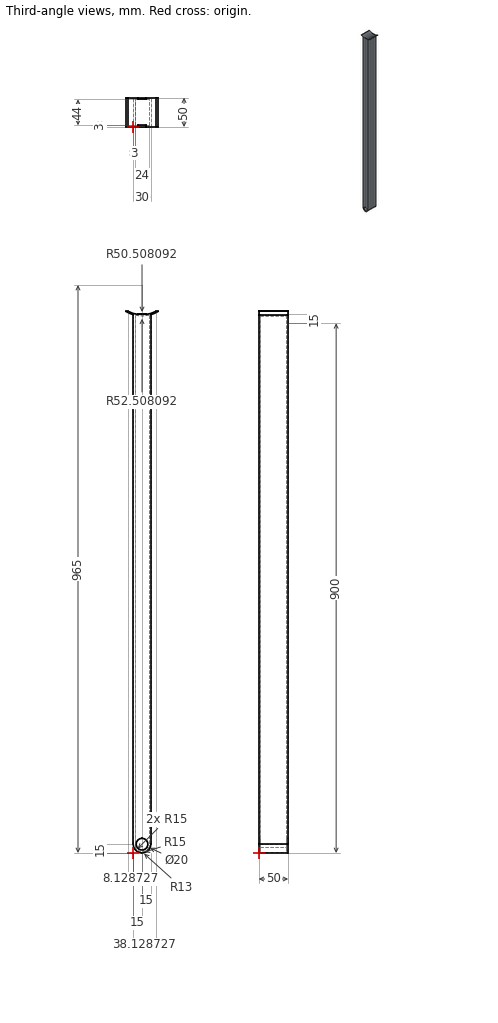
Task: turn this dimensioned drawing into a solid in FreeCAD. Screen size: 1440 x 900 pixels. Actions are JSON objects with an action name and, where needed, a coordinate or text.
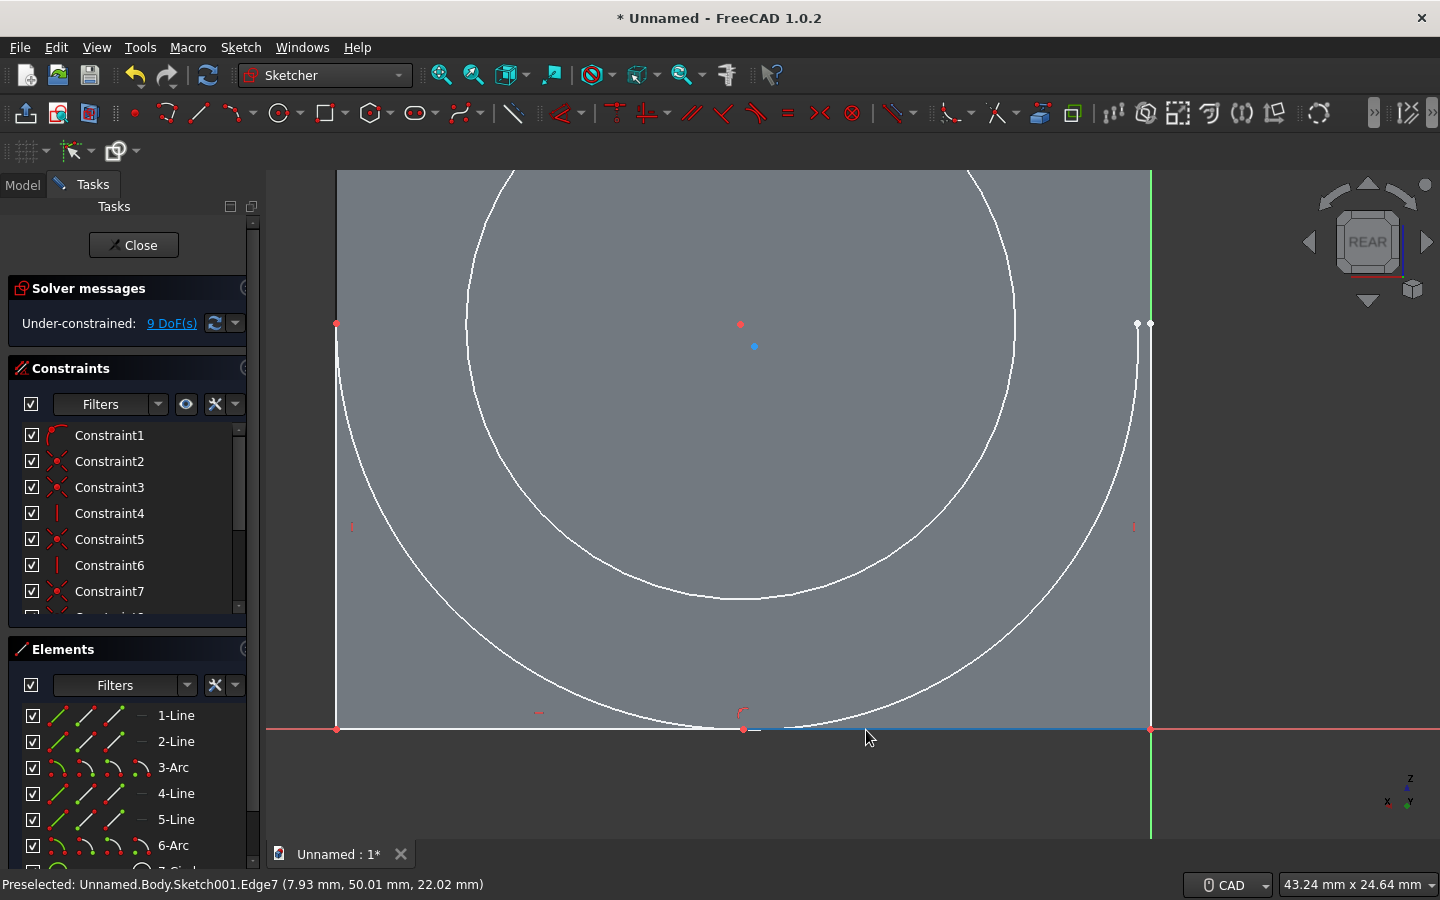
{"action": "left_click", "coordinate": [866, 729]}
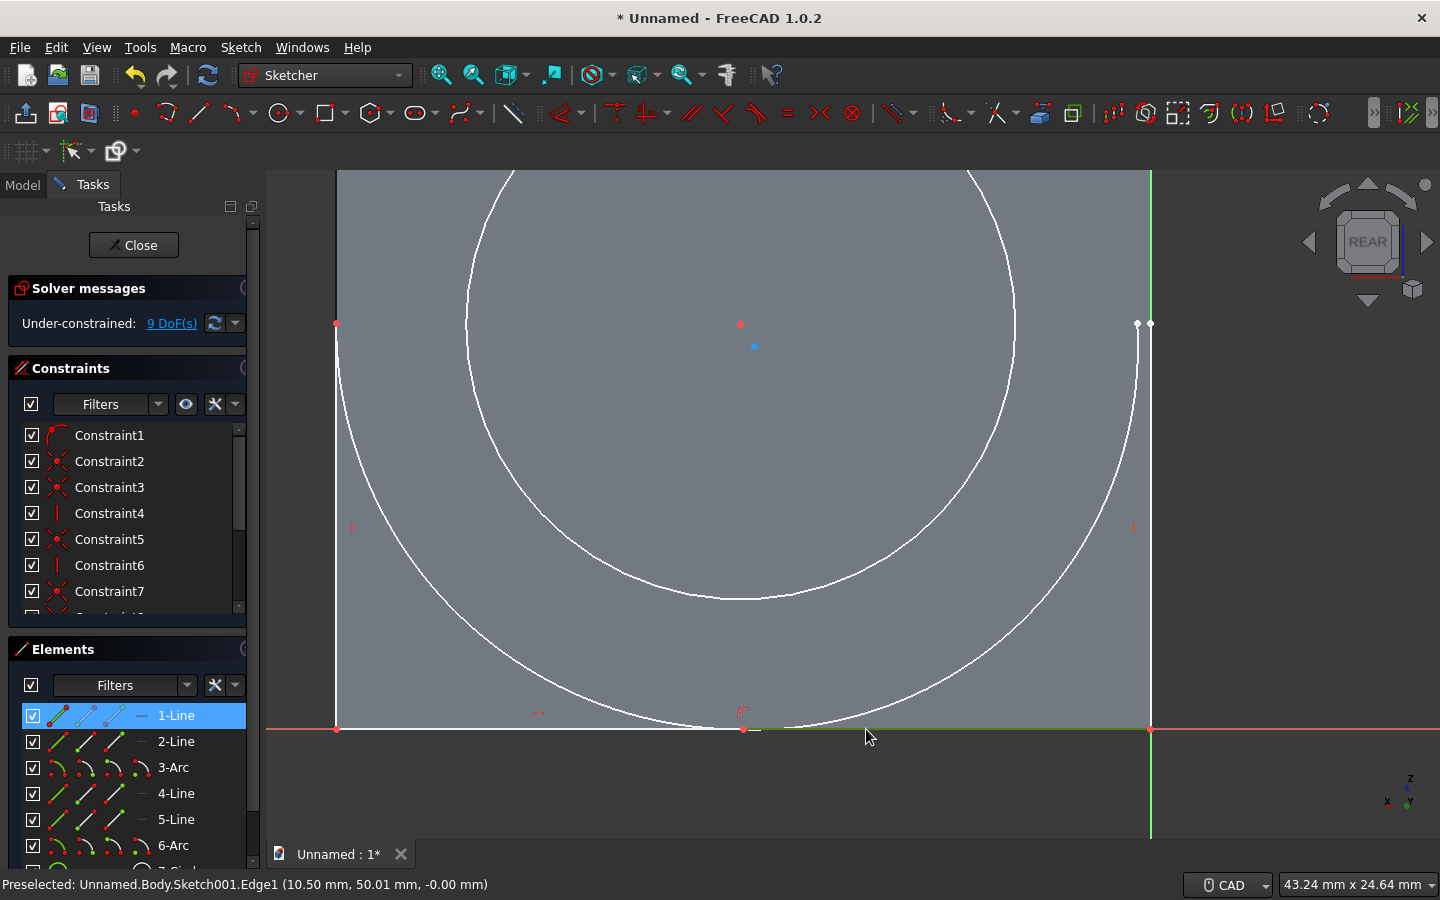
{"action": "left_click", "coordinate": [928, 688]}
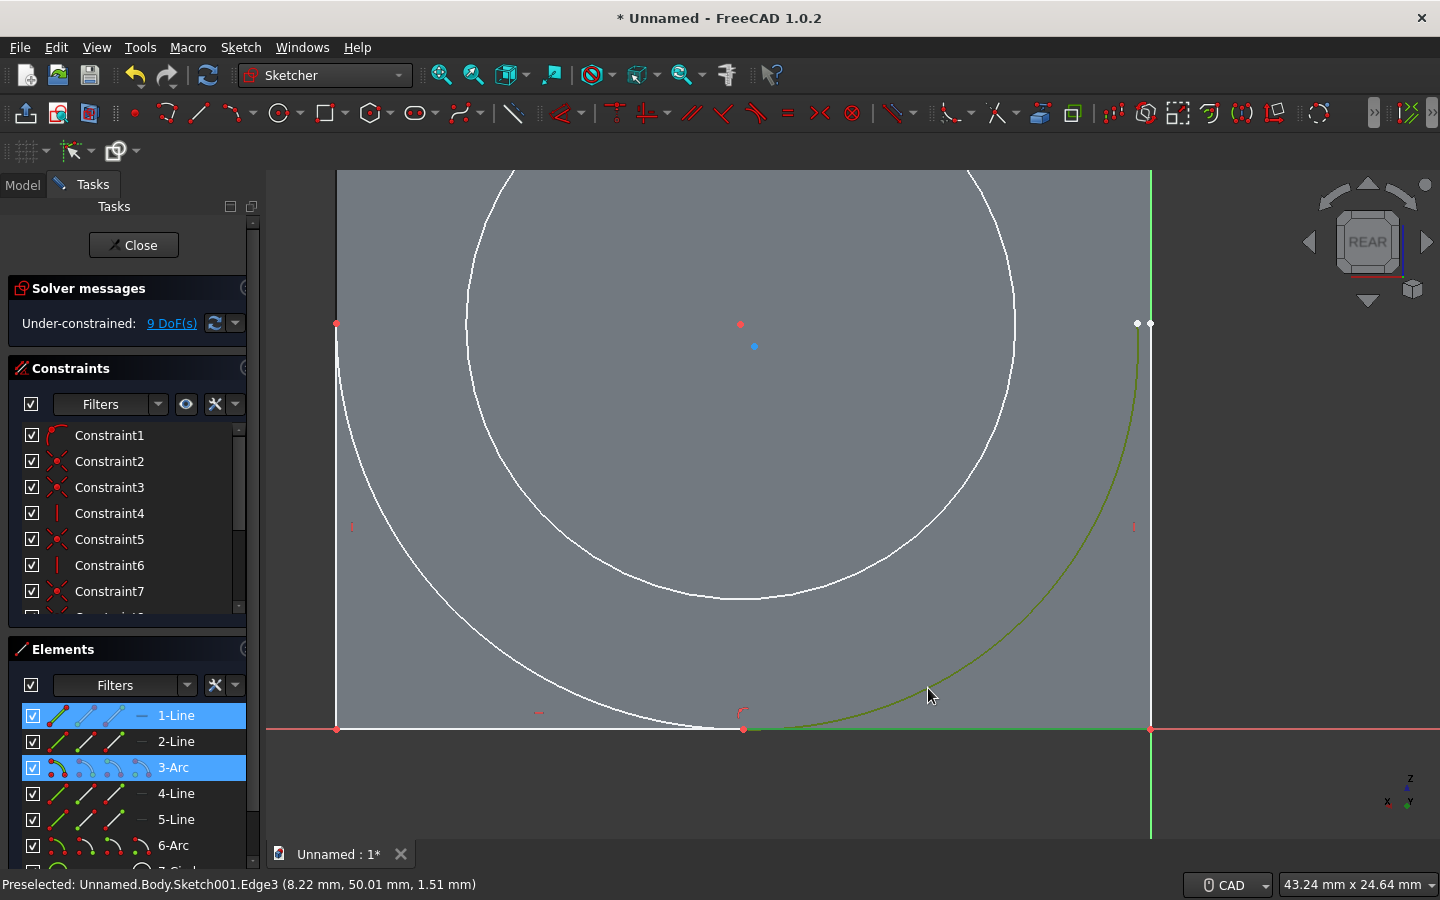
{"action": "left_click", "coordinate": [756, 114]}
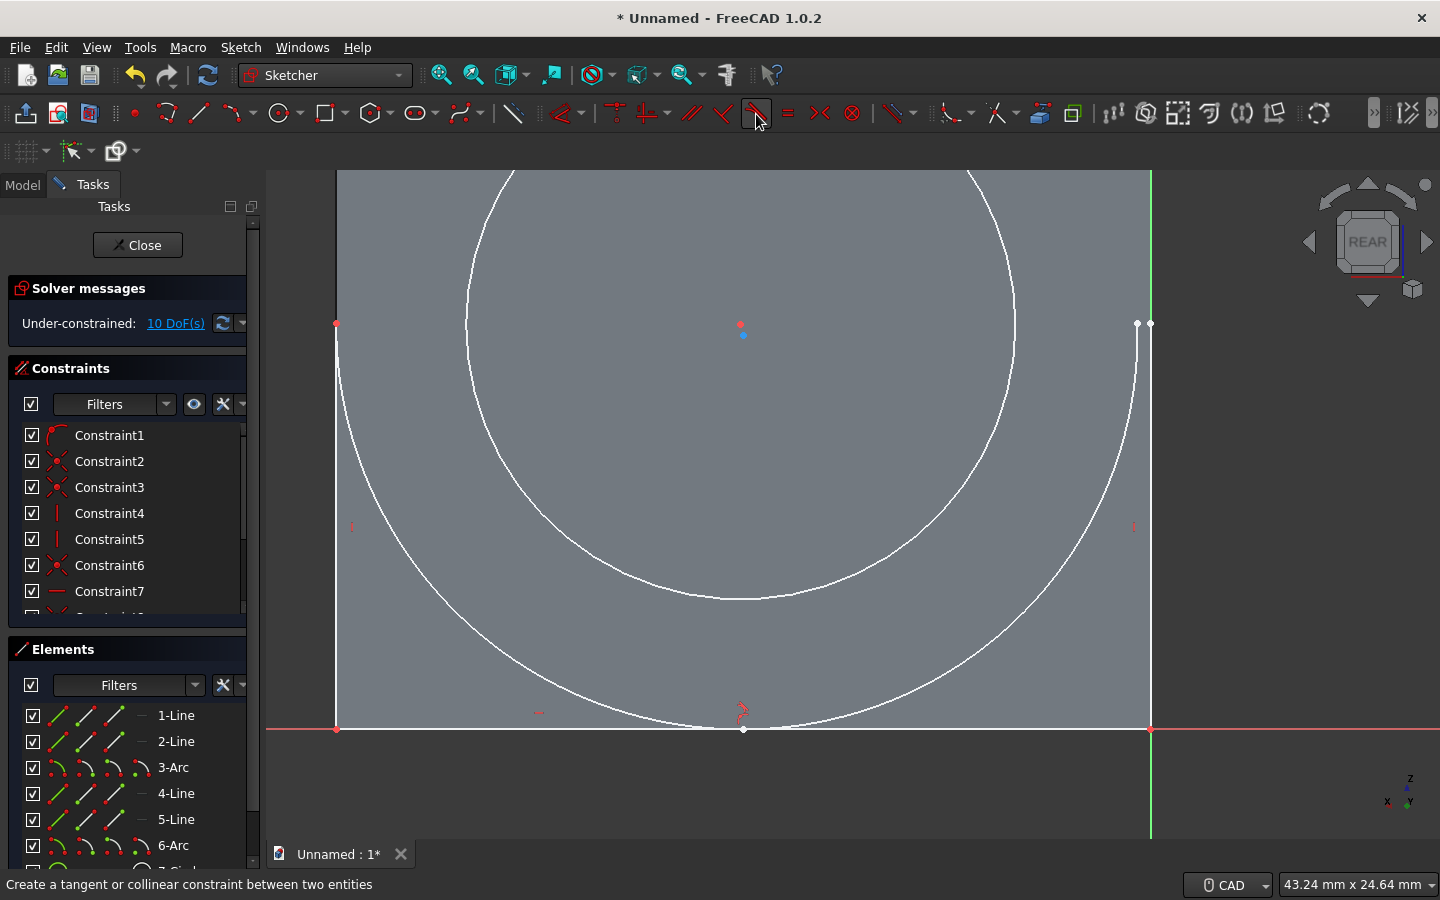
{"action": "left_click", "coordinate": [866, 729]}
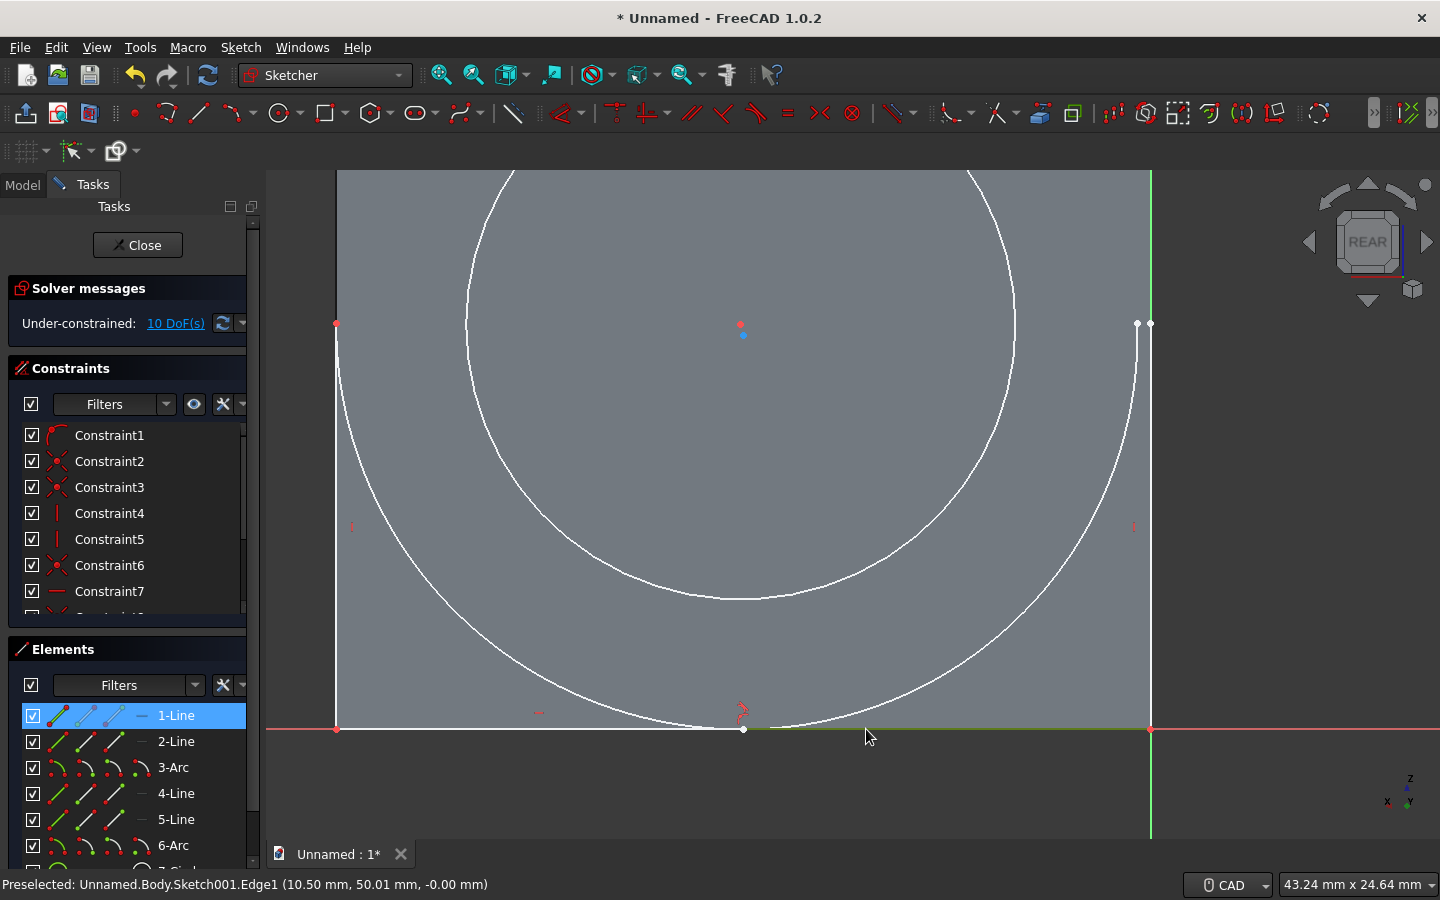
{"action": "left_click", "coordinate": [380, 509]}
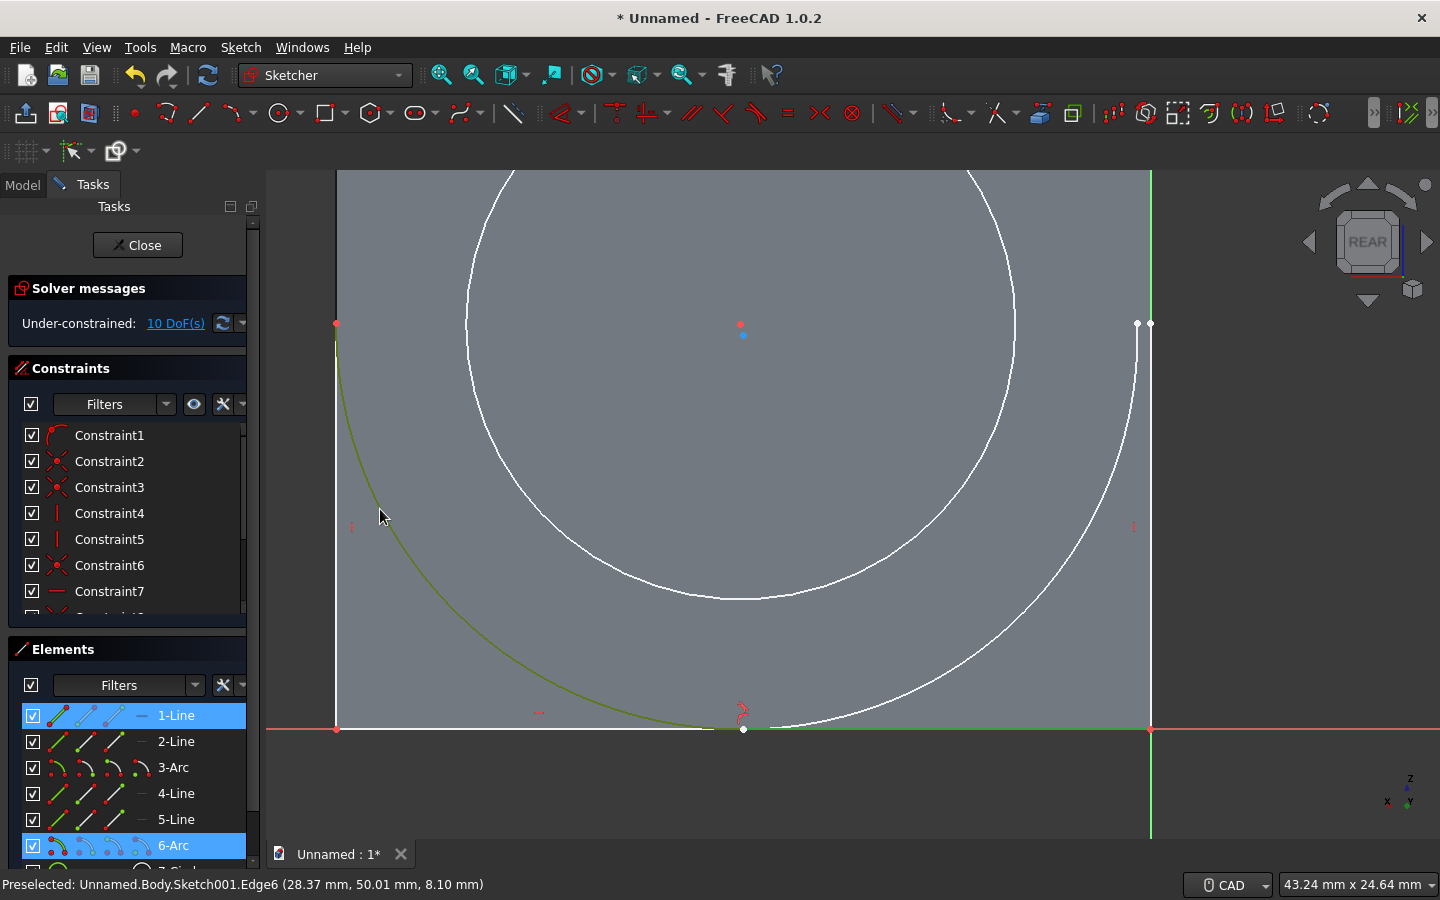
{"action": "left_click", "coordinate": [756, 114]}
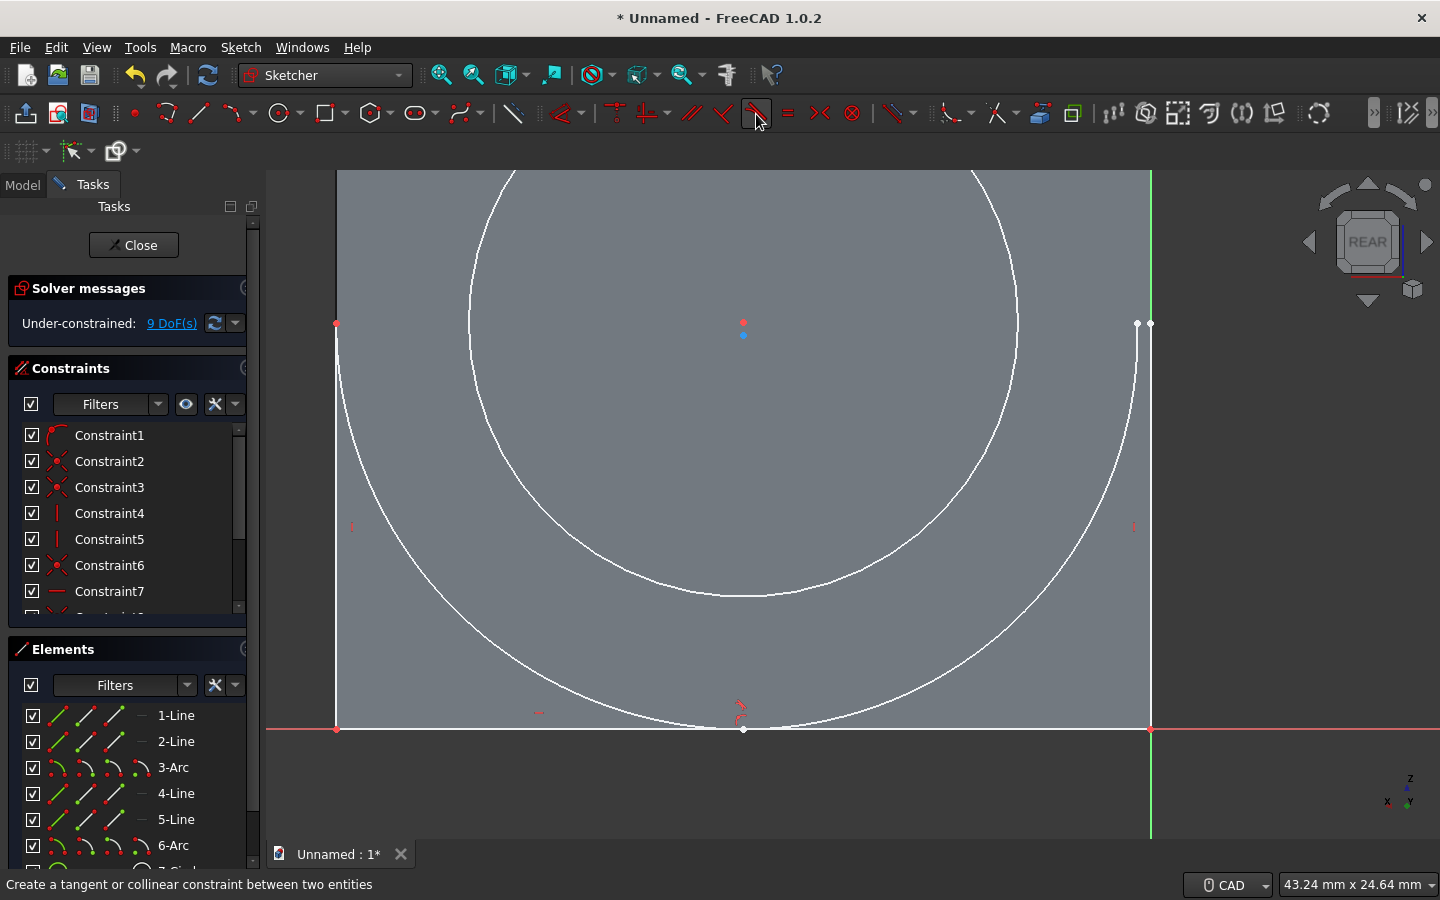
{"action": "left_click", "coordinate": [1151, 608]}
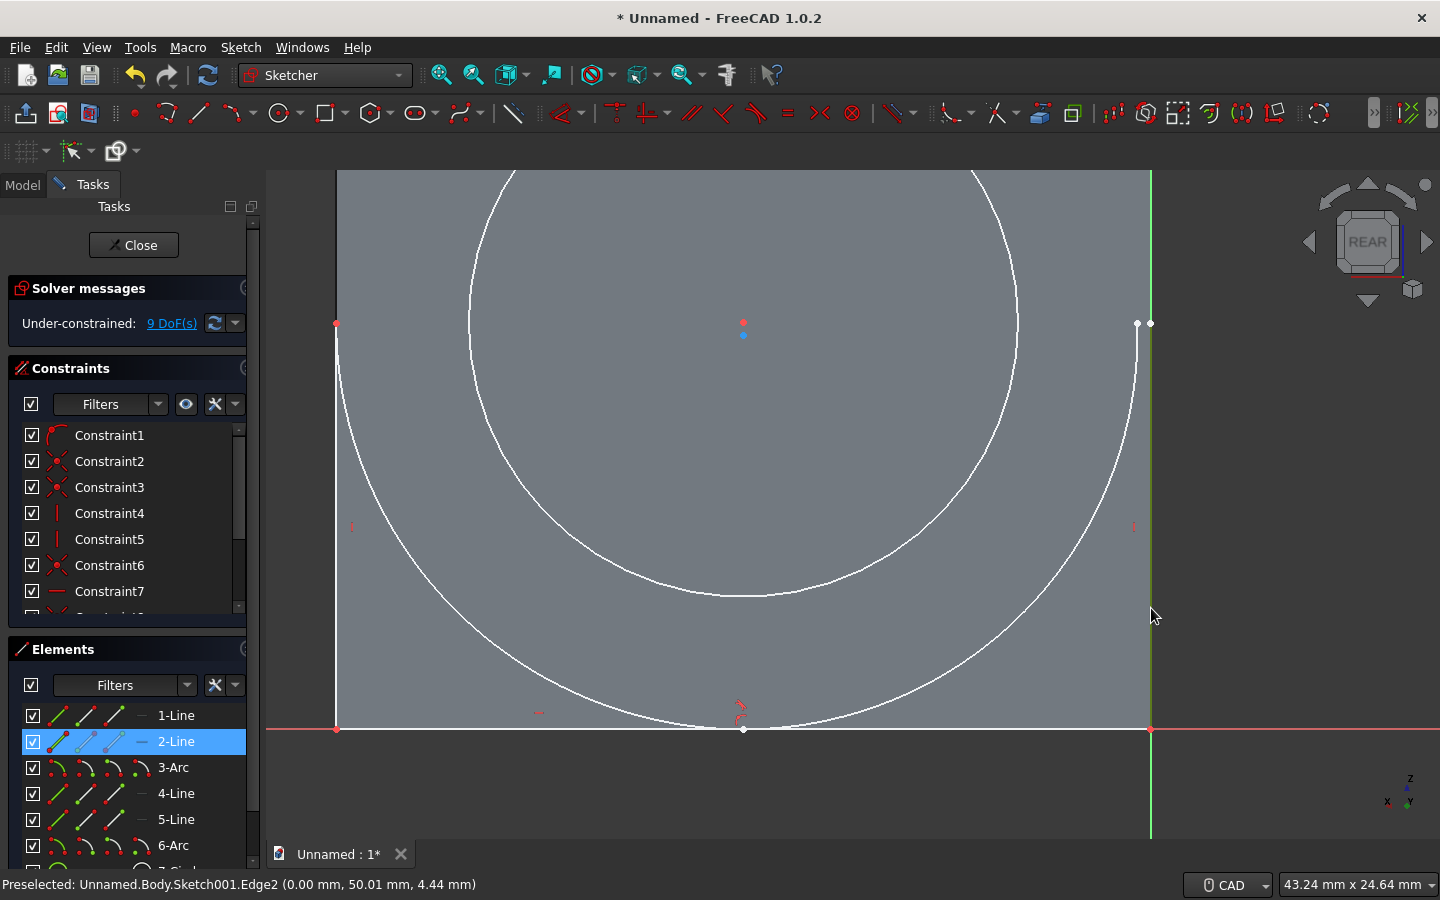
{"action": "left_click", "coordinate": [925, 685]}